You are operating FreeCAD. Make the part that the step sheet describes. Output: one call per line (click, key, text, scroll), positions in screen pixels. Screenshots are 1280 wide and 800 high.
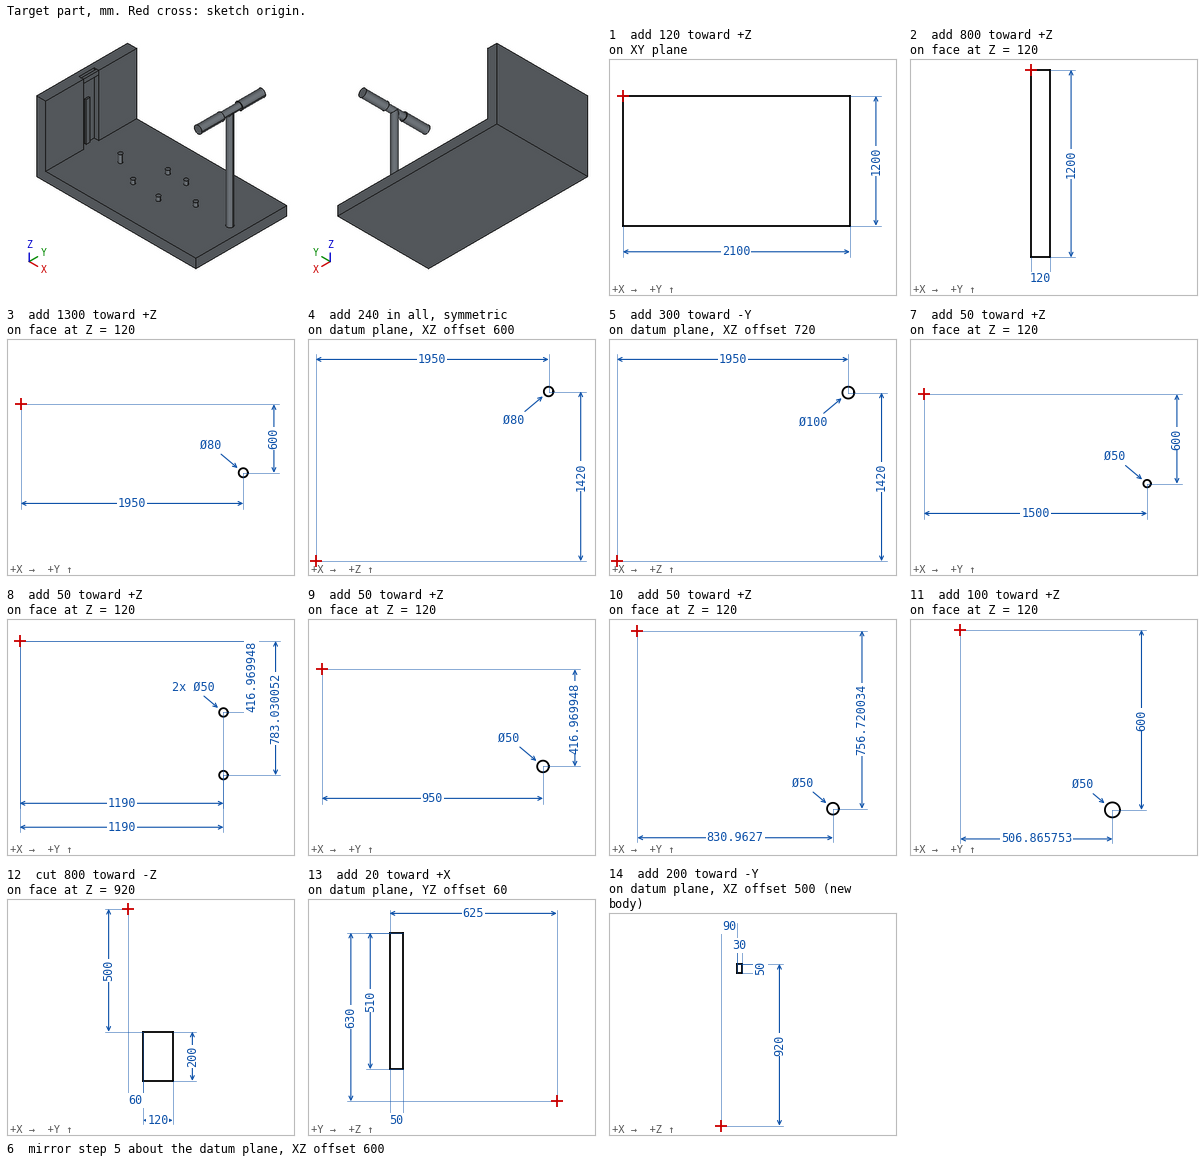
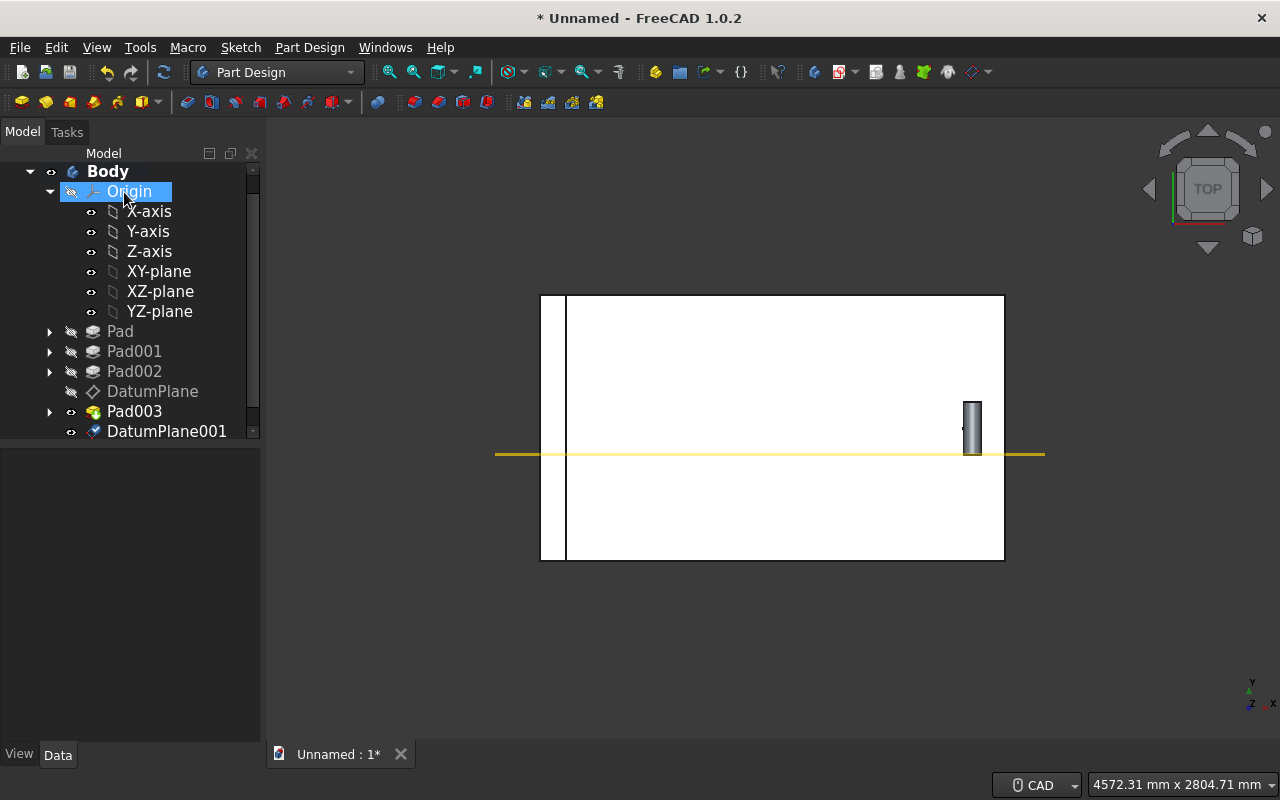
click(116, 432)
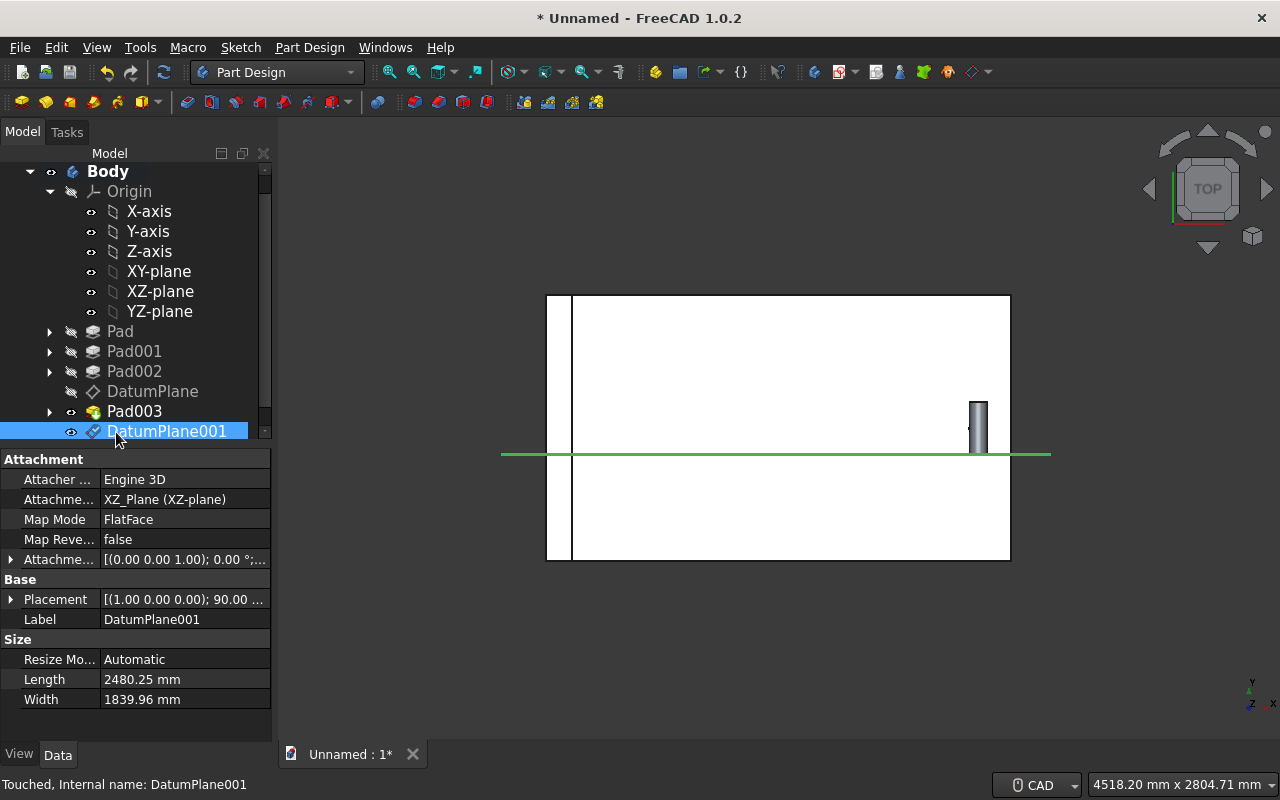
click(840, 72)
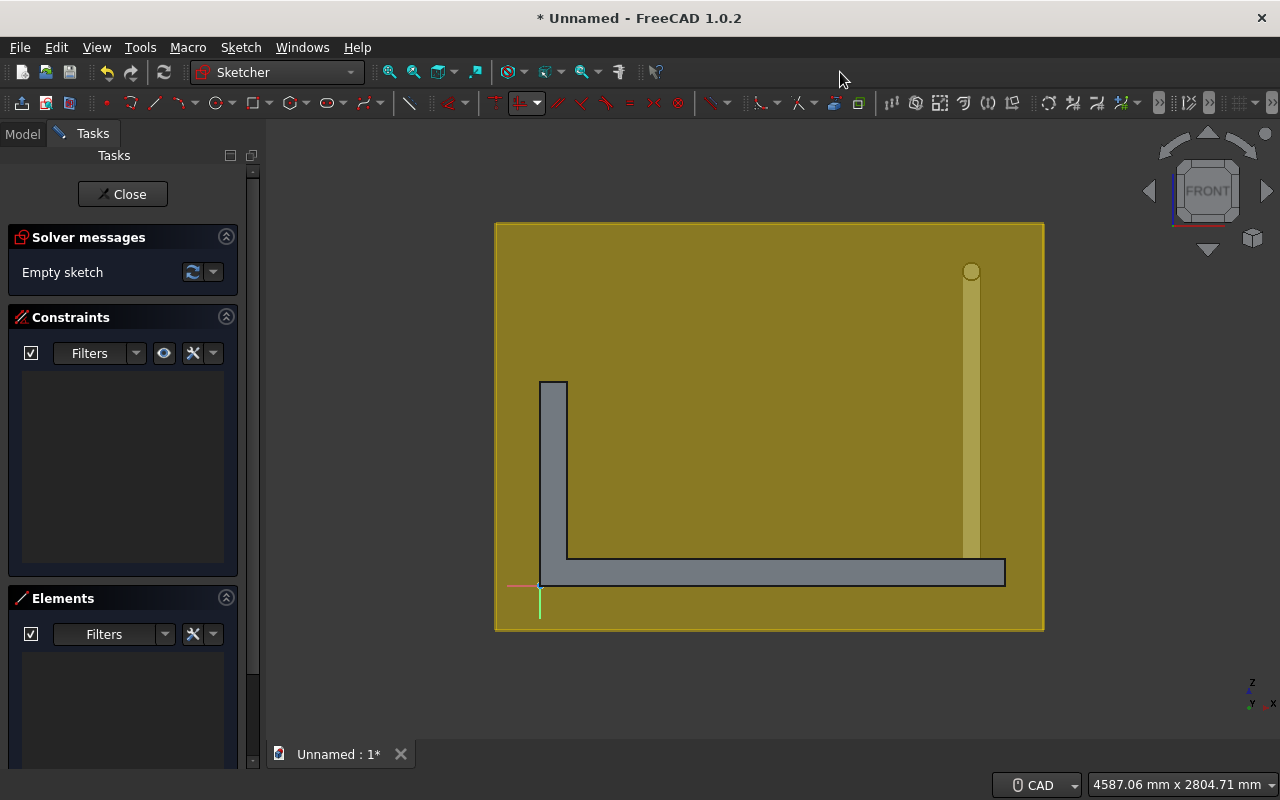
click(70, 104)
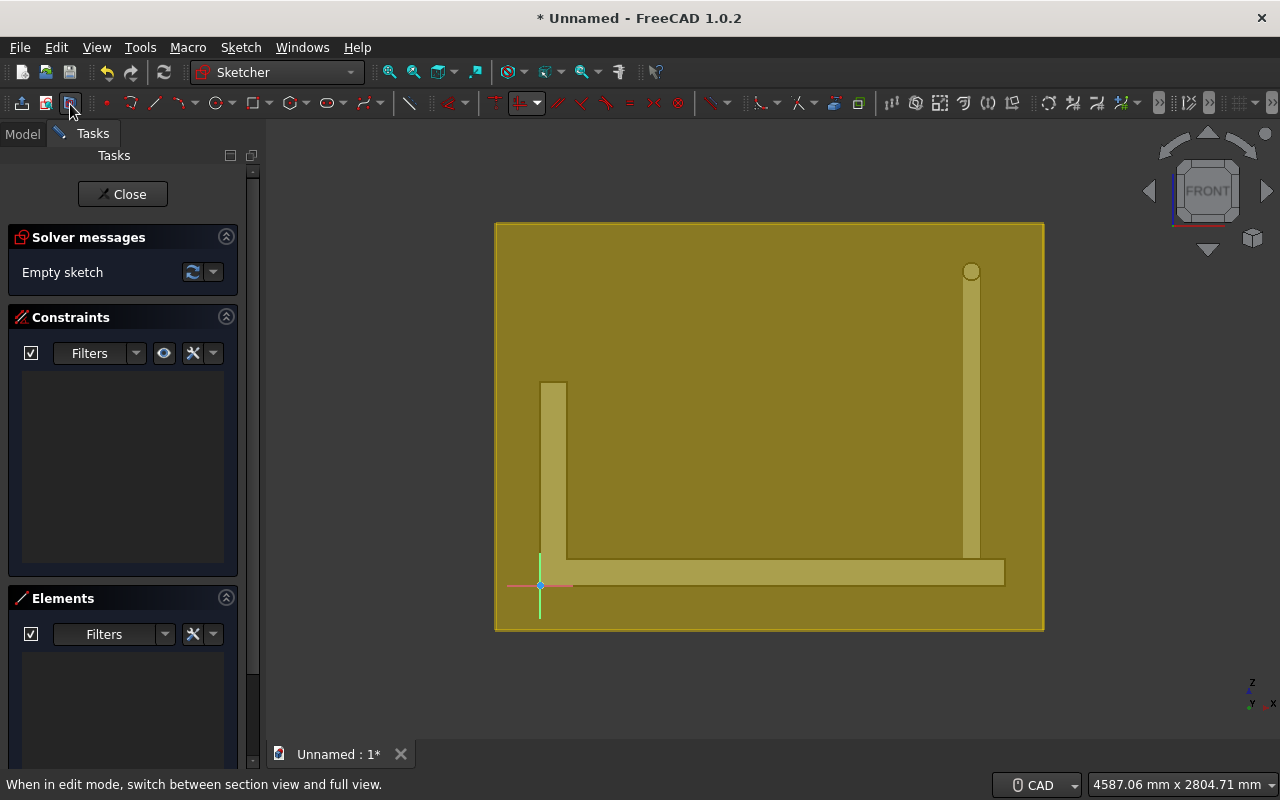
scroll(989, 261, up, 14)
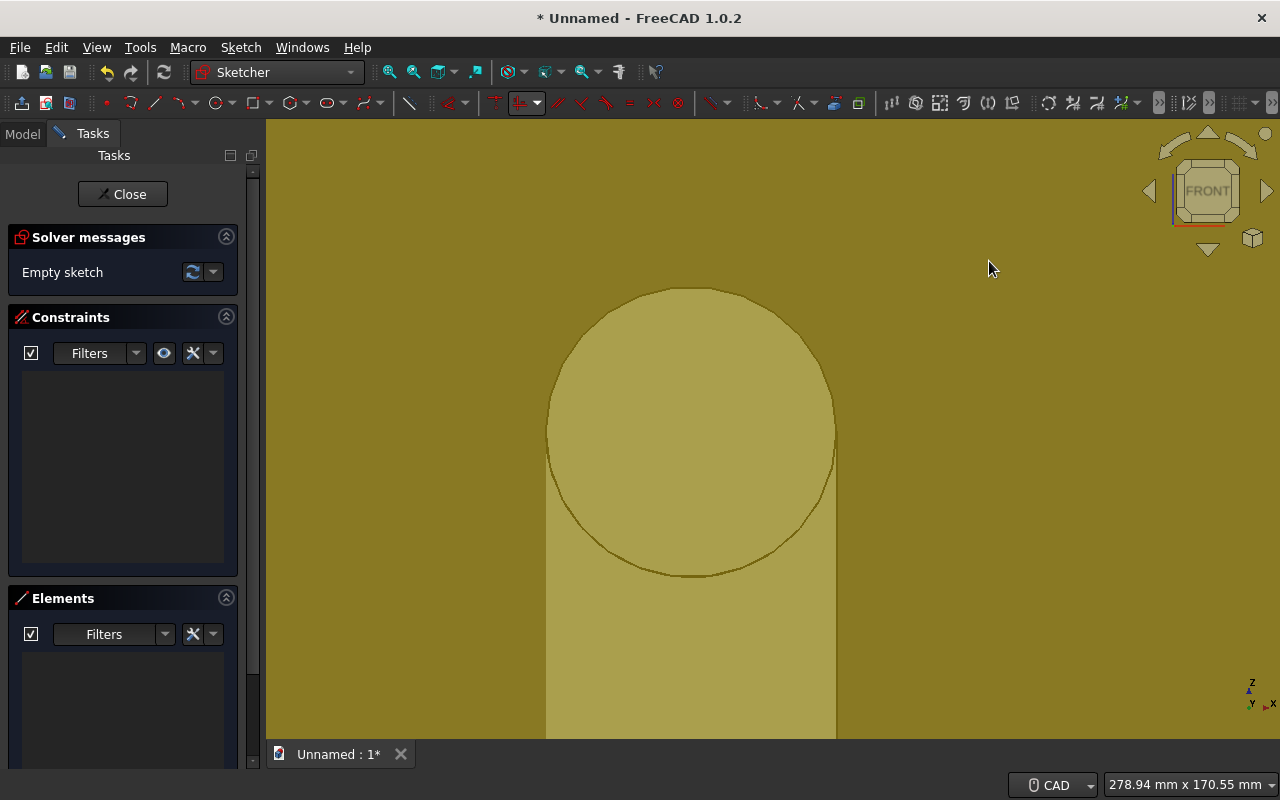
key(g)
key(c)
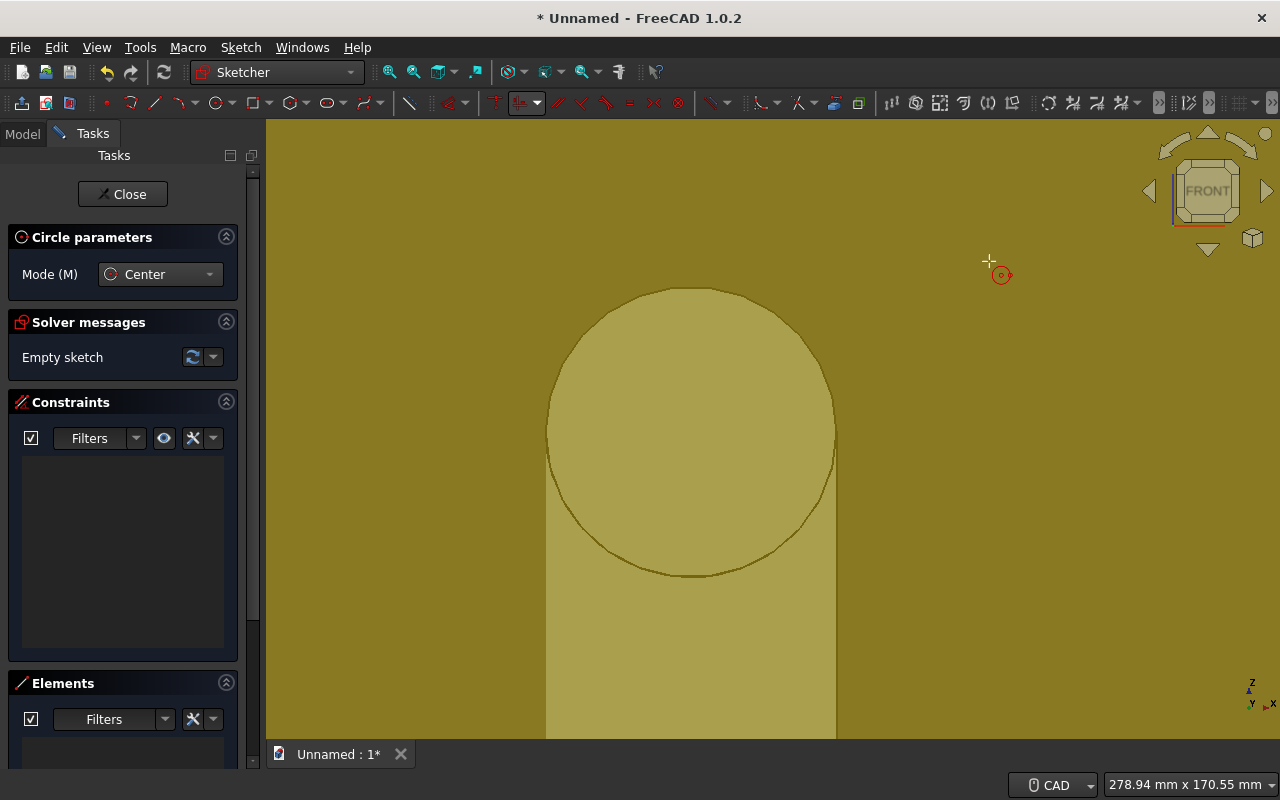
click(691, 432)
move(820, 303)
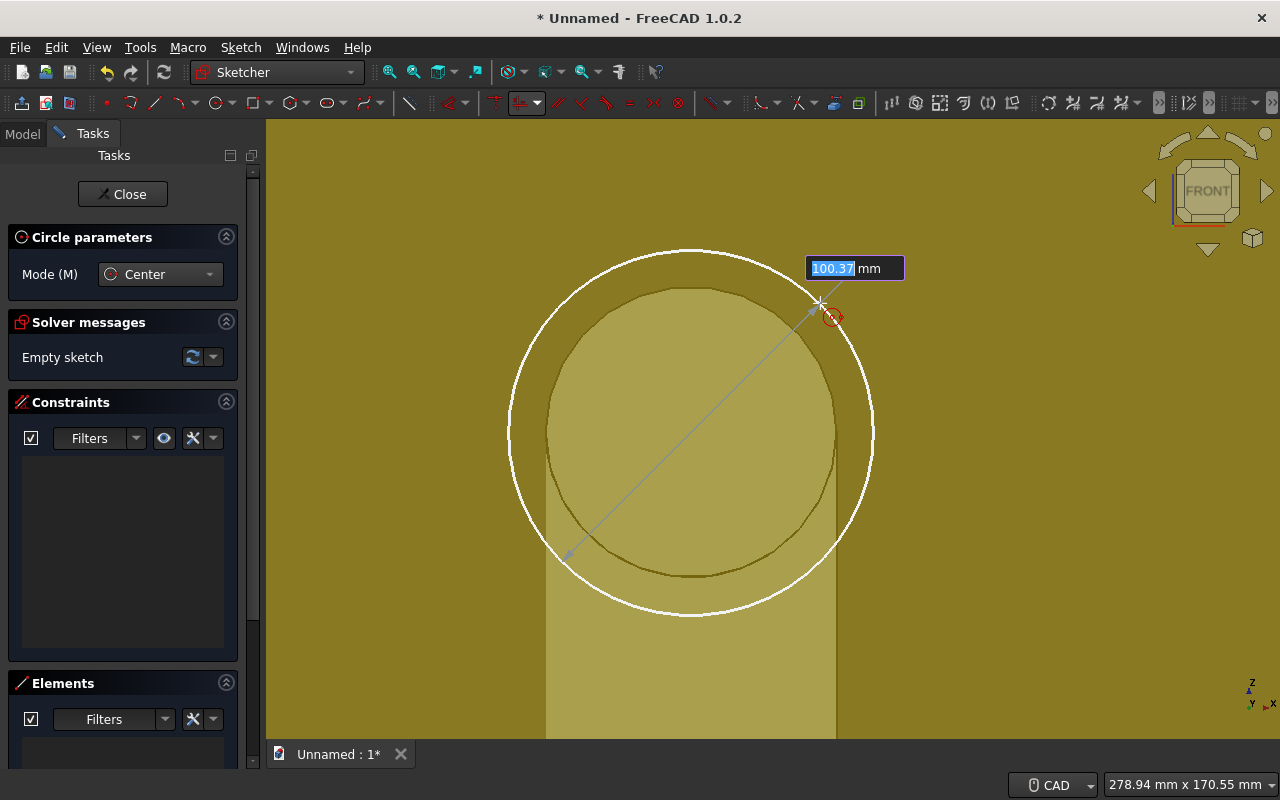
text(100)
key(Return)
key(Escape)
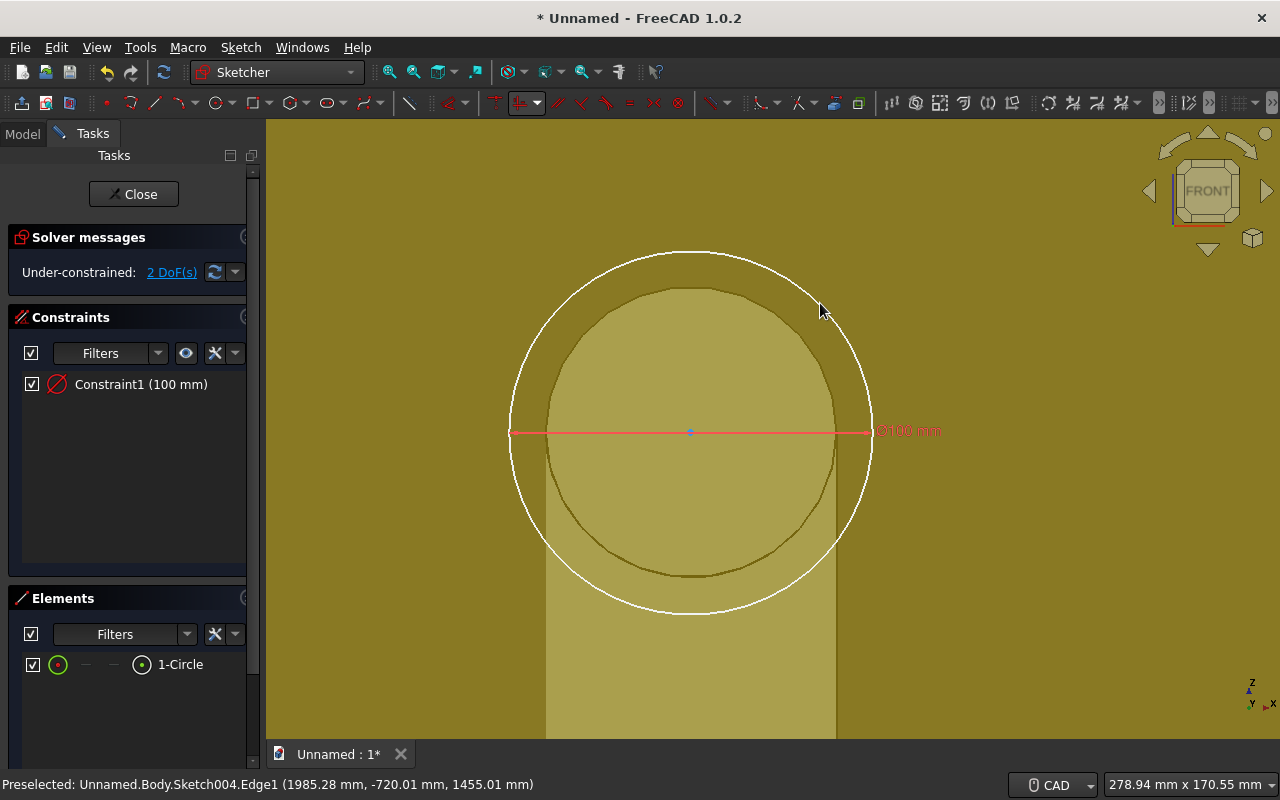
click(448, 104)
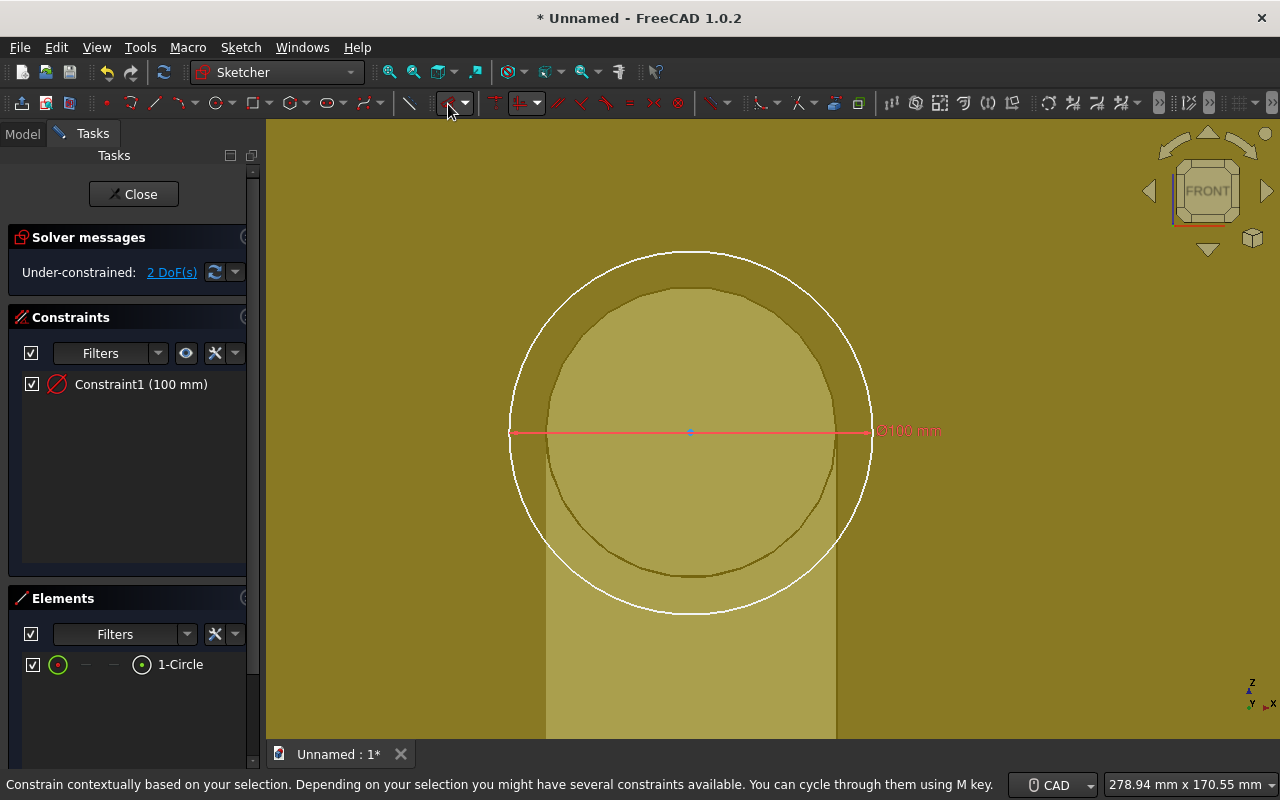
click(691, 433)
click(492, 399)